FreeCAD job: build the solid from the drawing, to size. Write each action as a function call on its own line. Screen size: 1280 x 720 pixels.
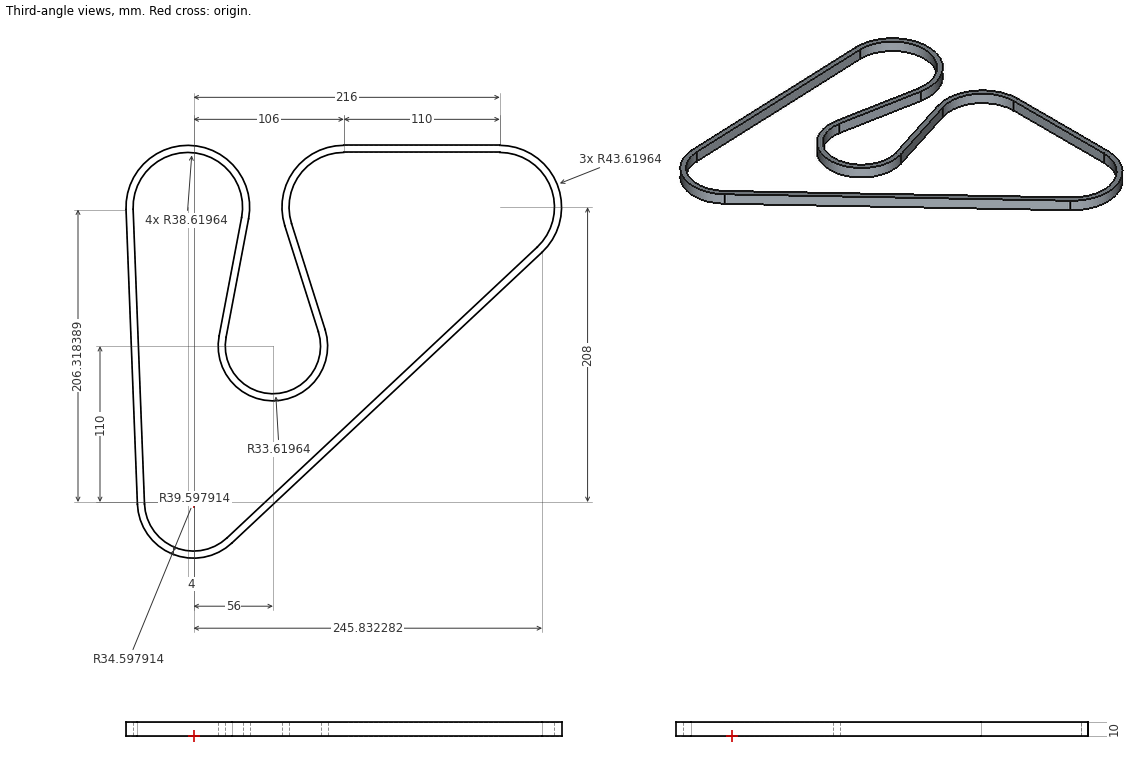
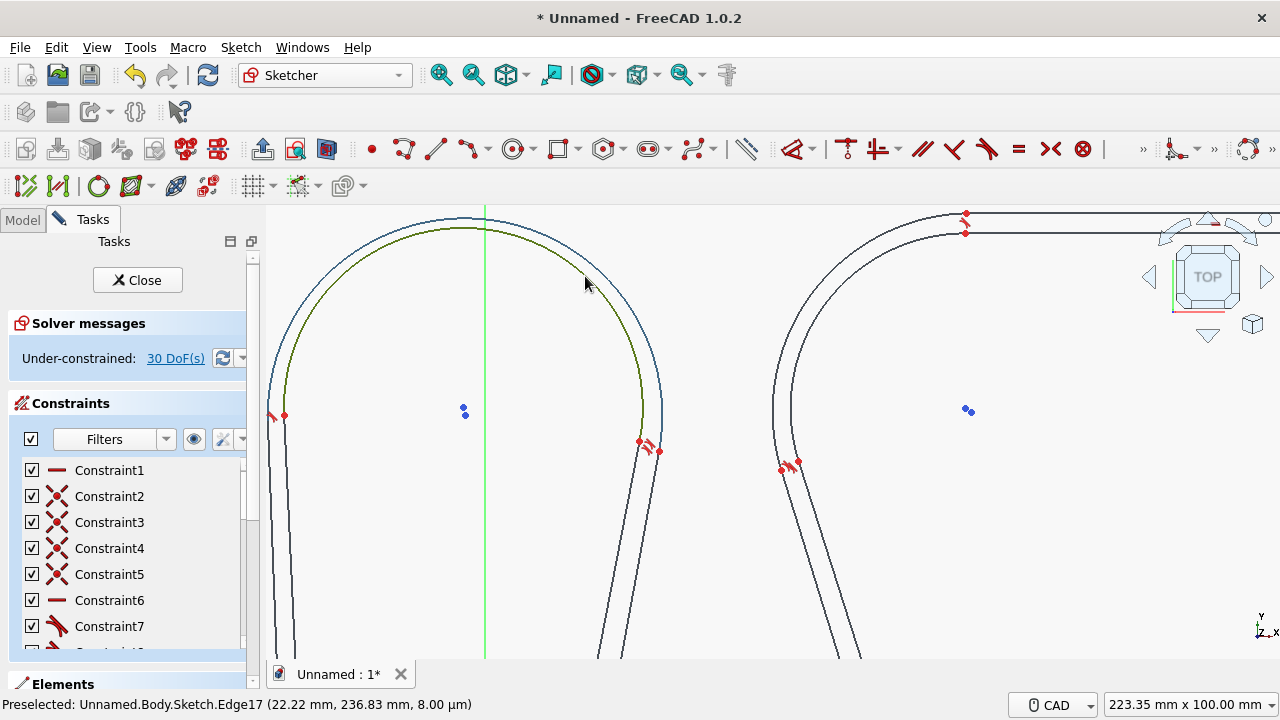
click(846, 150)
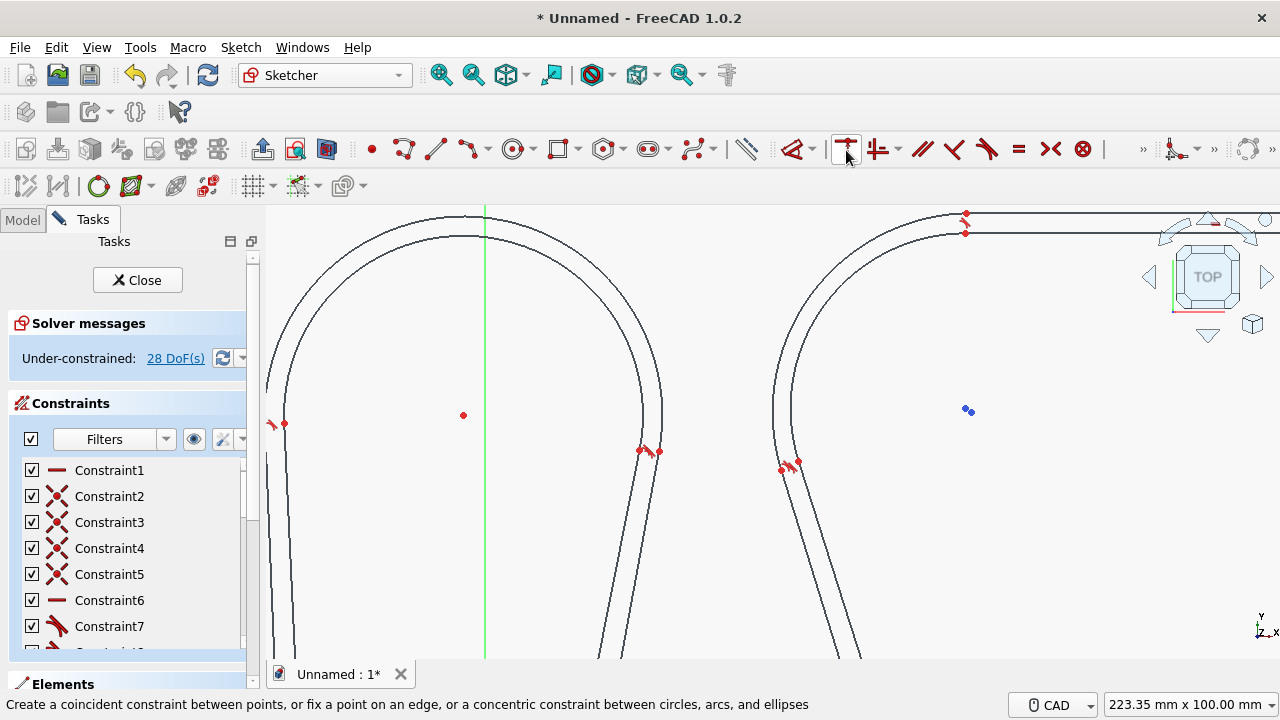
scroll(640, 323, down, 8)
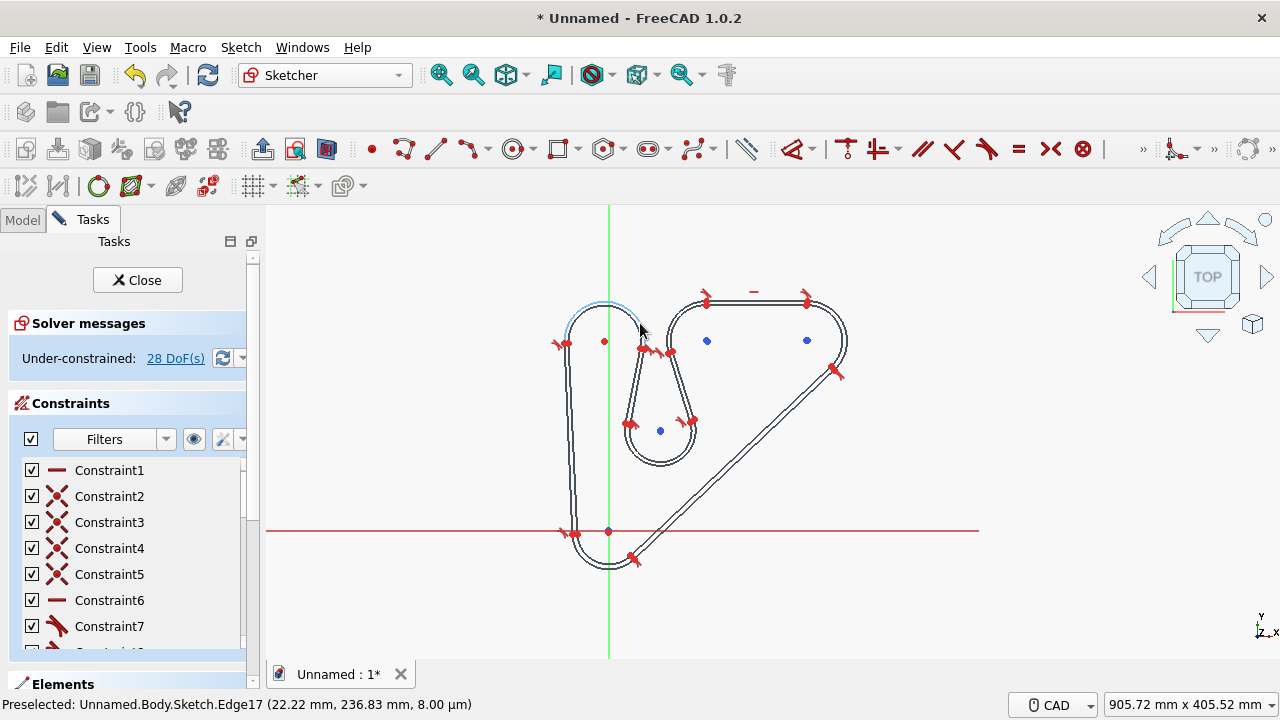
scroll(641, 456, up, 7)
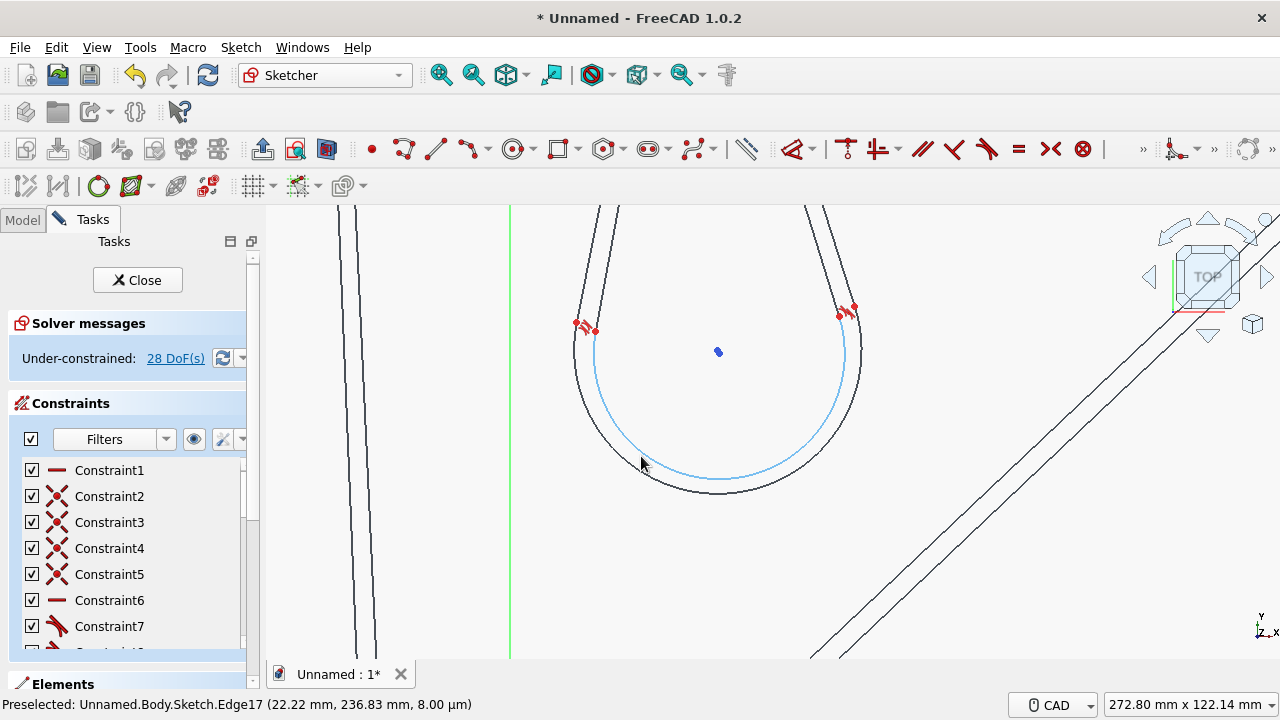
click(642, 452)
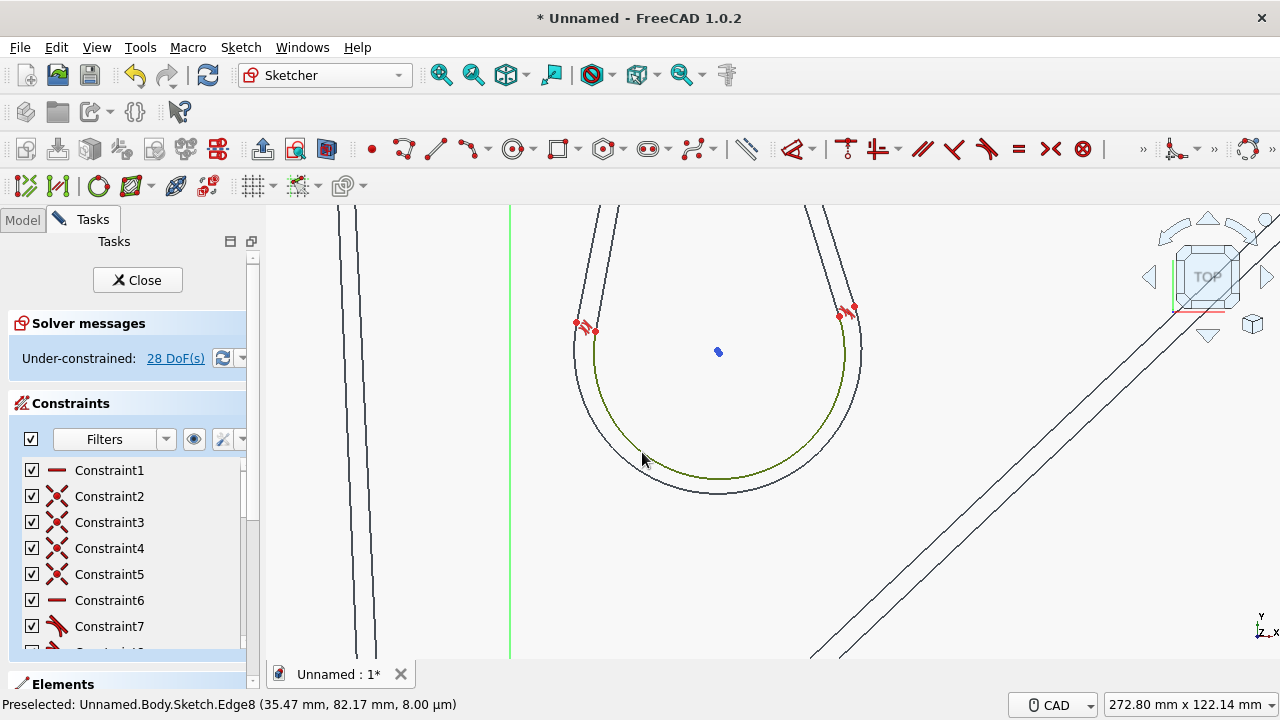
click(628, 463)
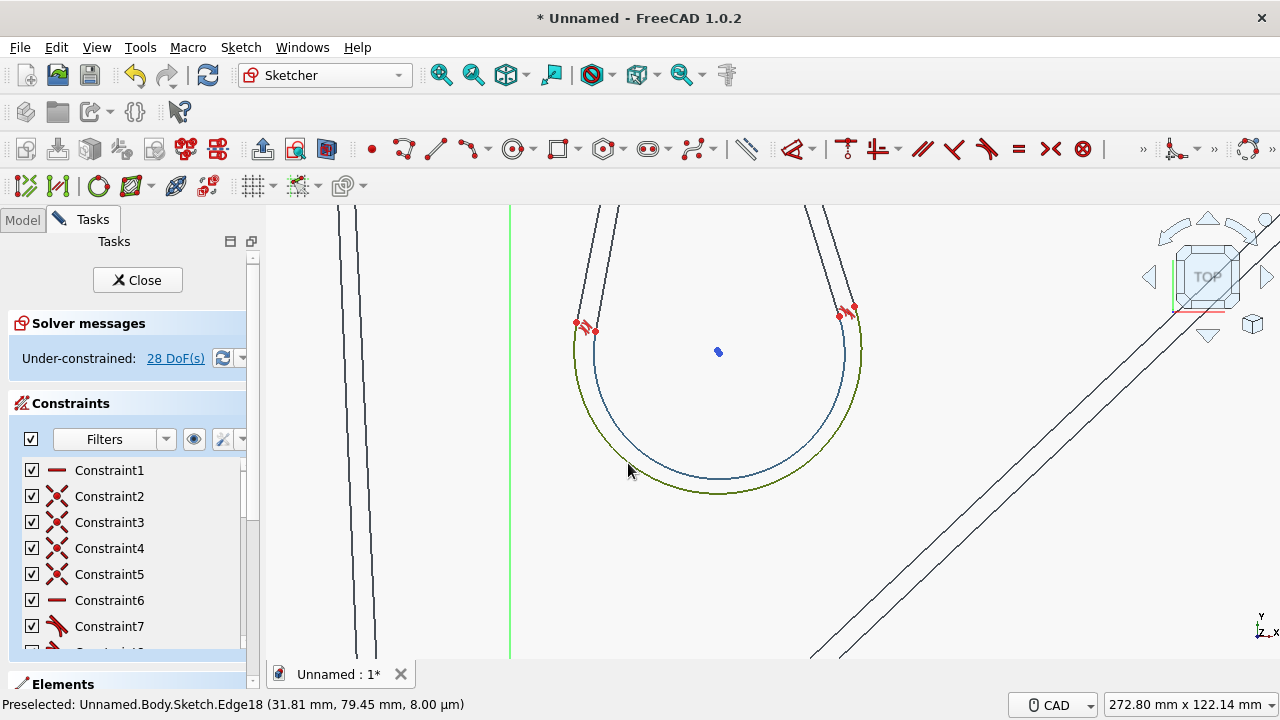
click(846, 150)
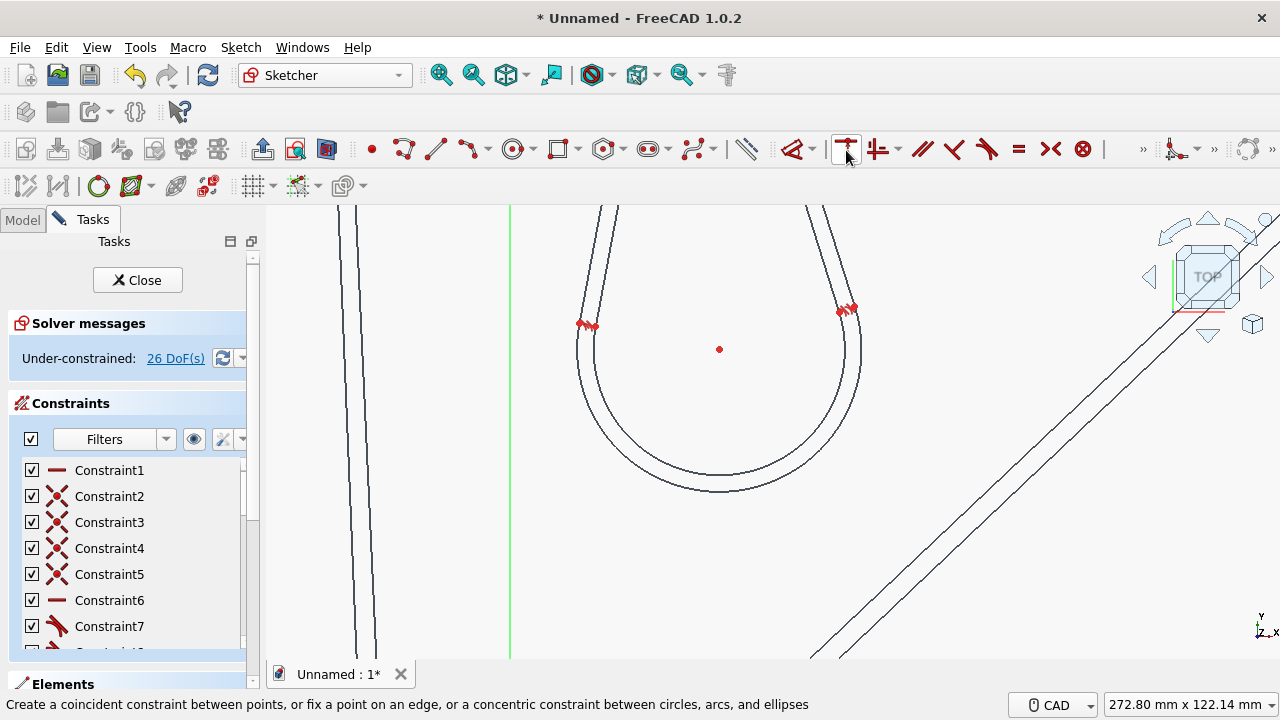
scroll(641, 456, down, 7)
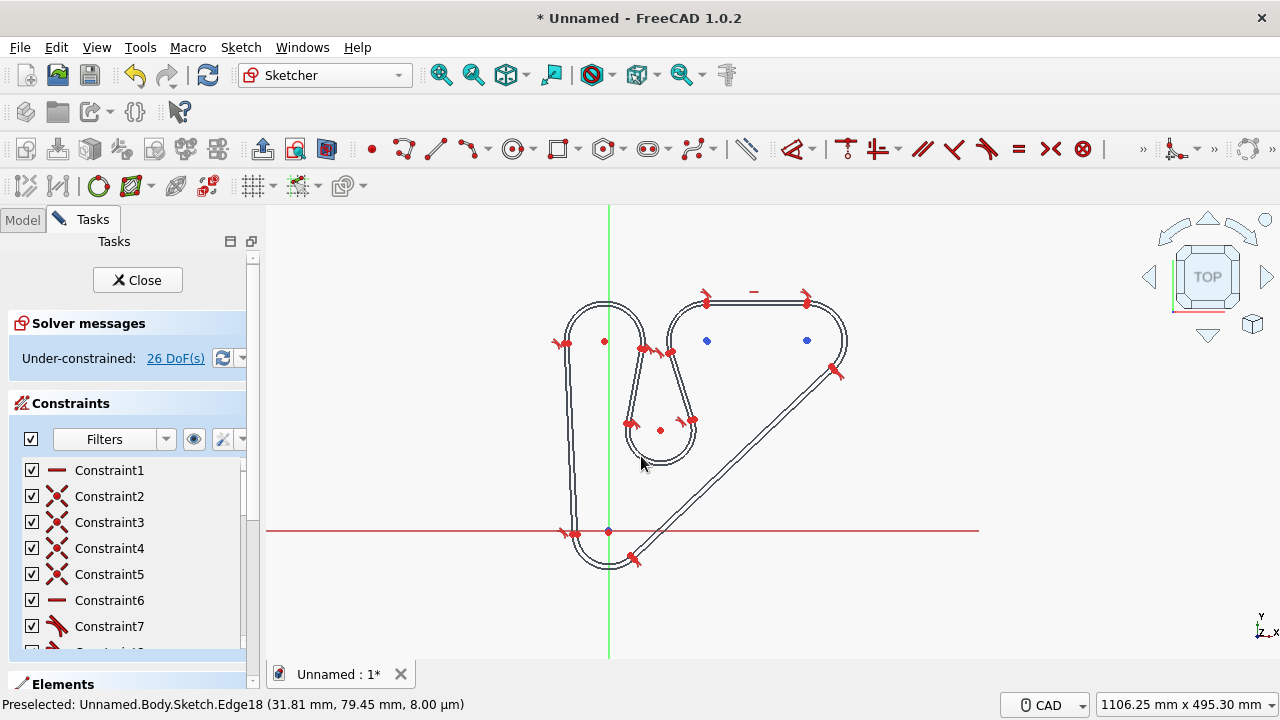
scroll(685, 308, up, 7)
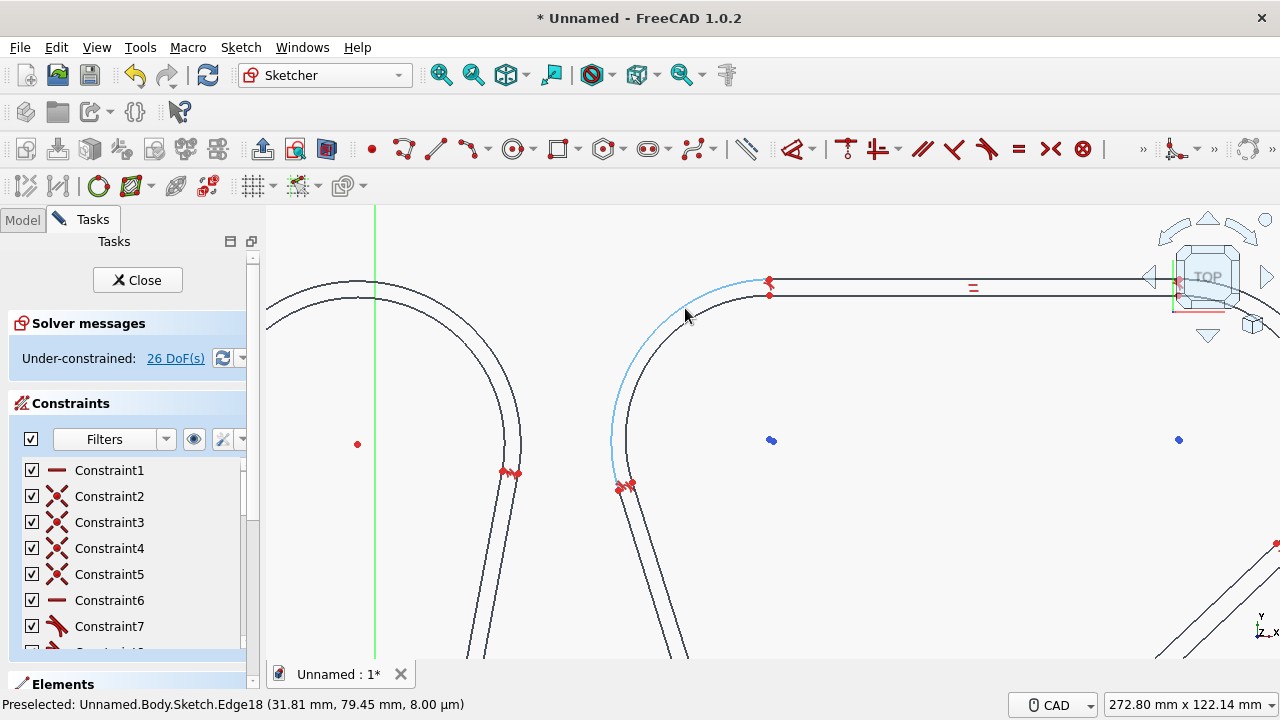
click(685, 306)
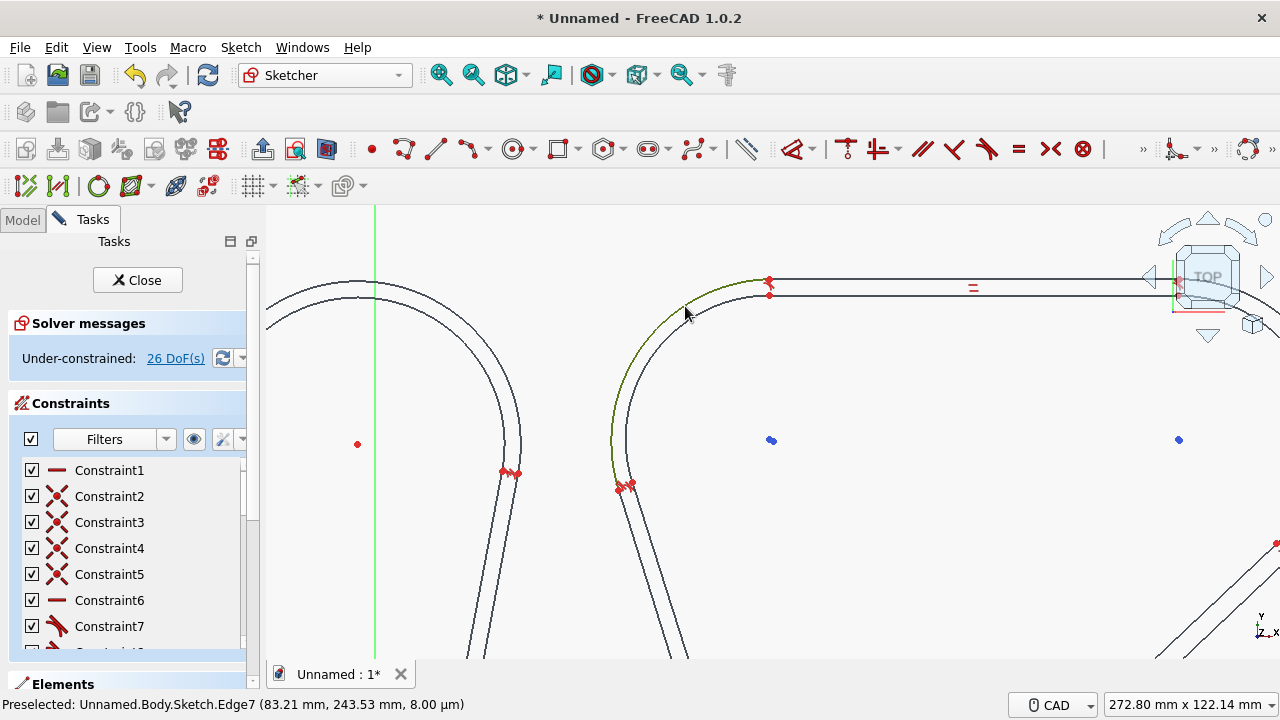
click(693, 318)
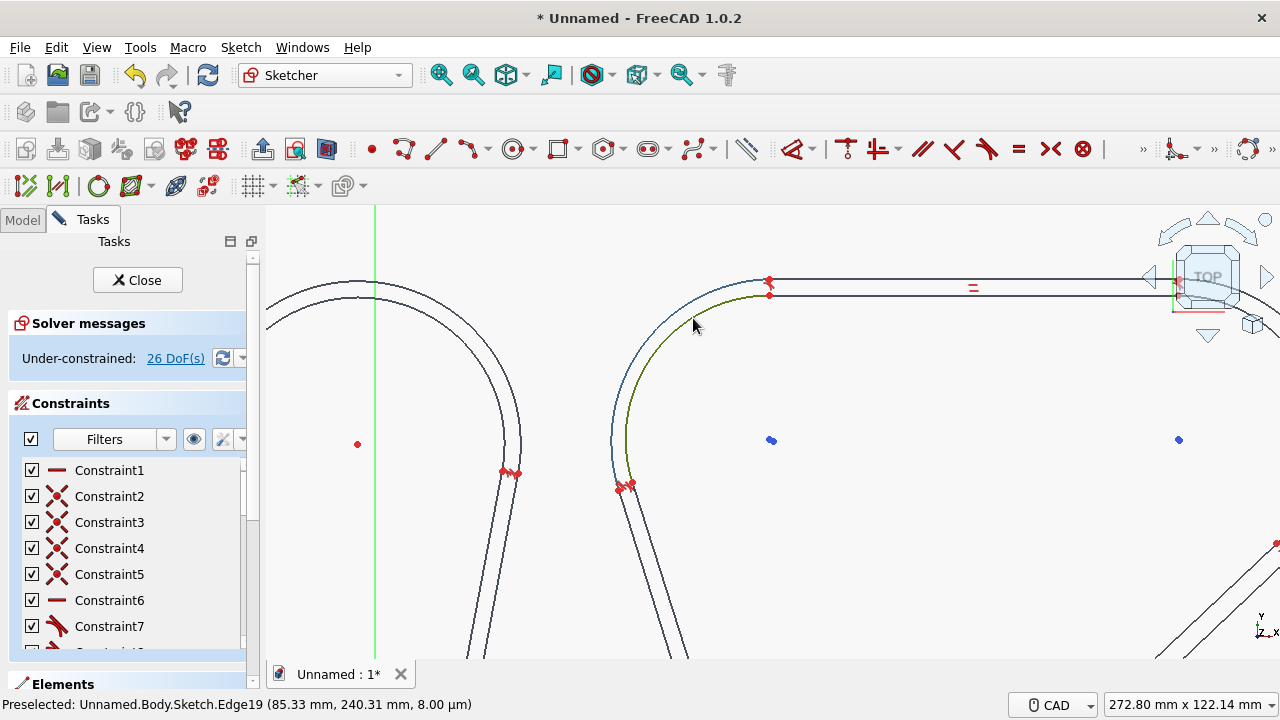
click(846, 150)